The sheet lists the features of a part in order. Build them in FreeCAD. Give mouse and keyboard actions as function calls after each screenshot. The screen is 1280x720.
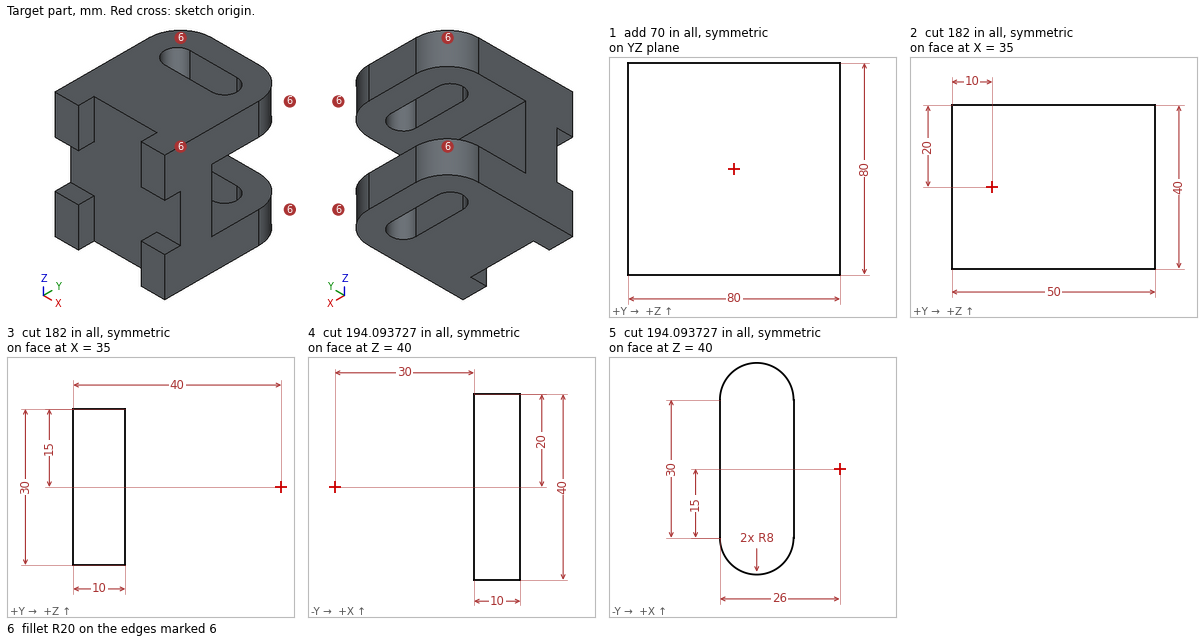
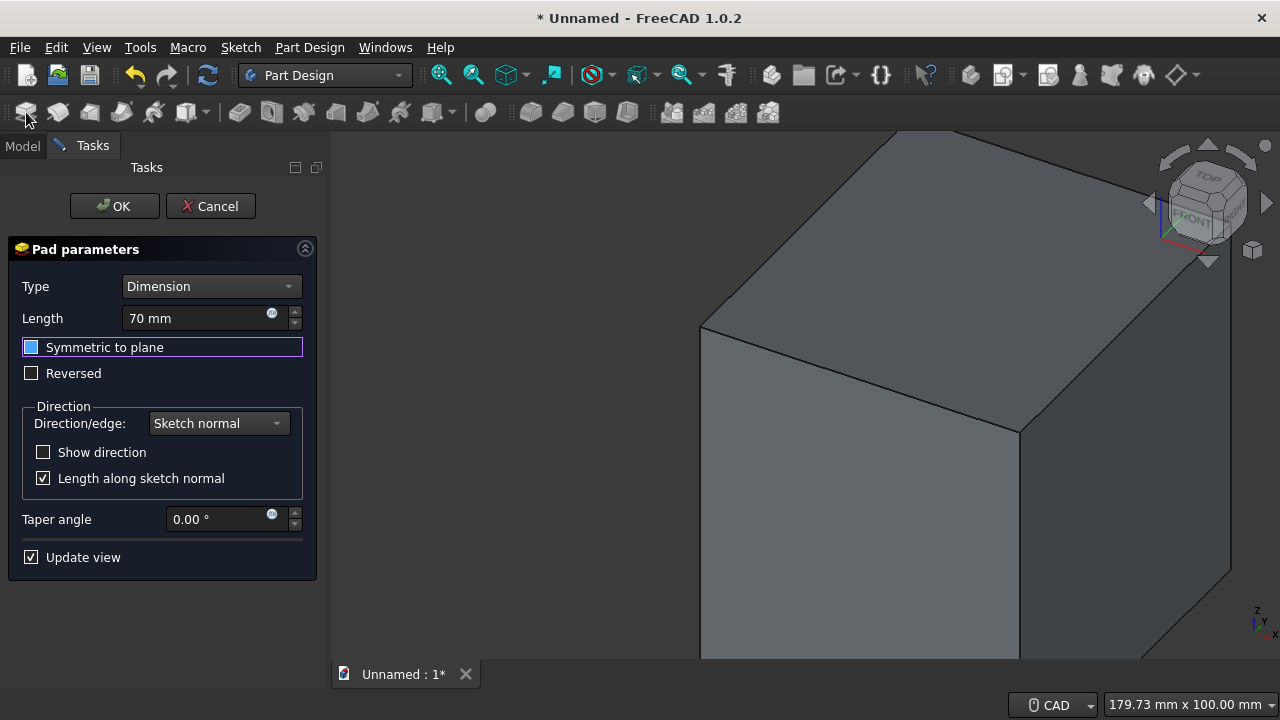
click(30, 347)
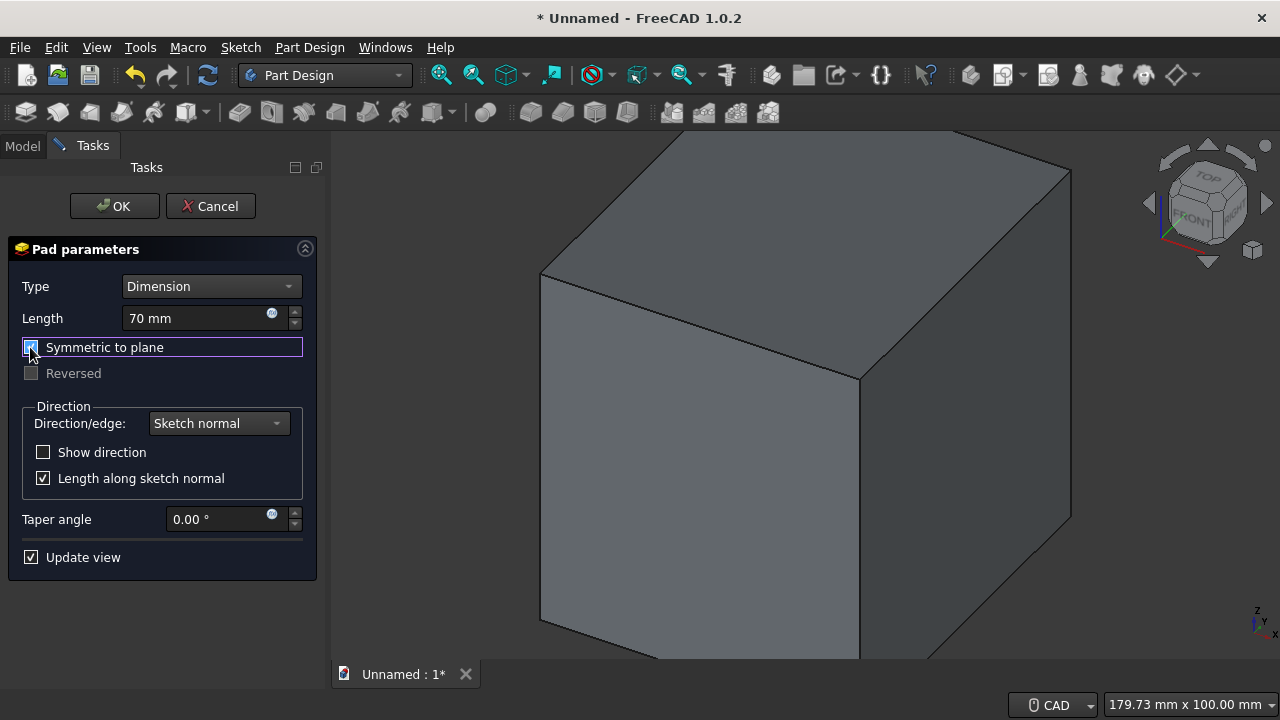
click(115, 206)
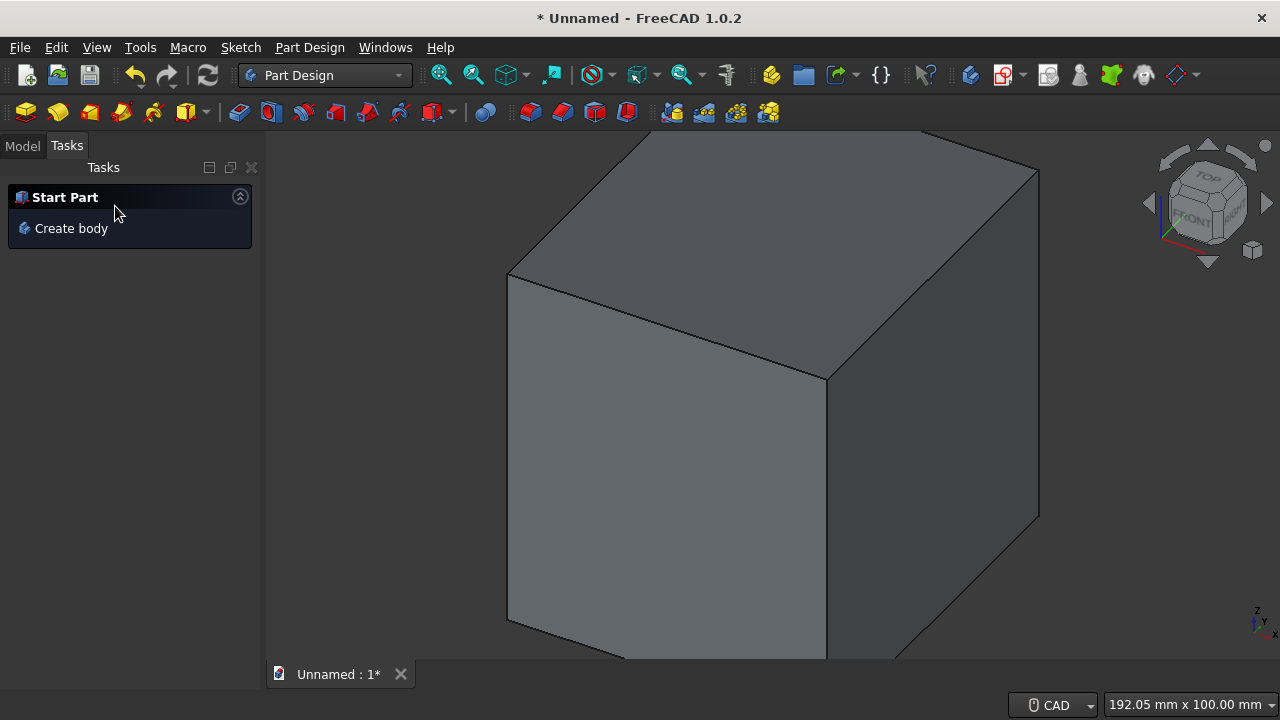
click(442, 76)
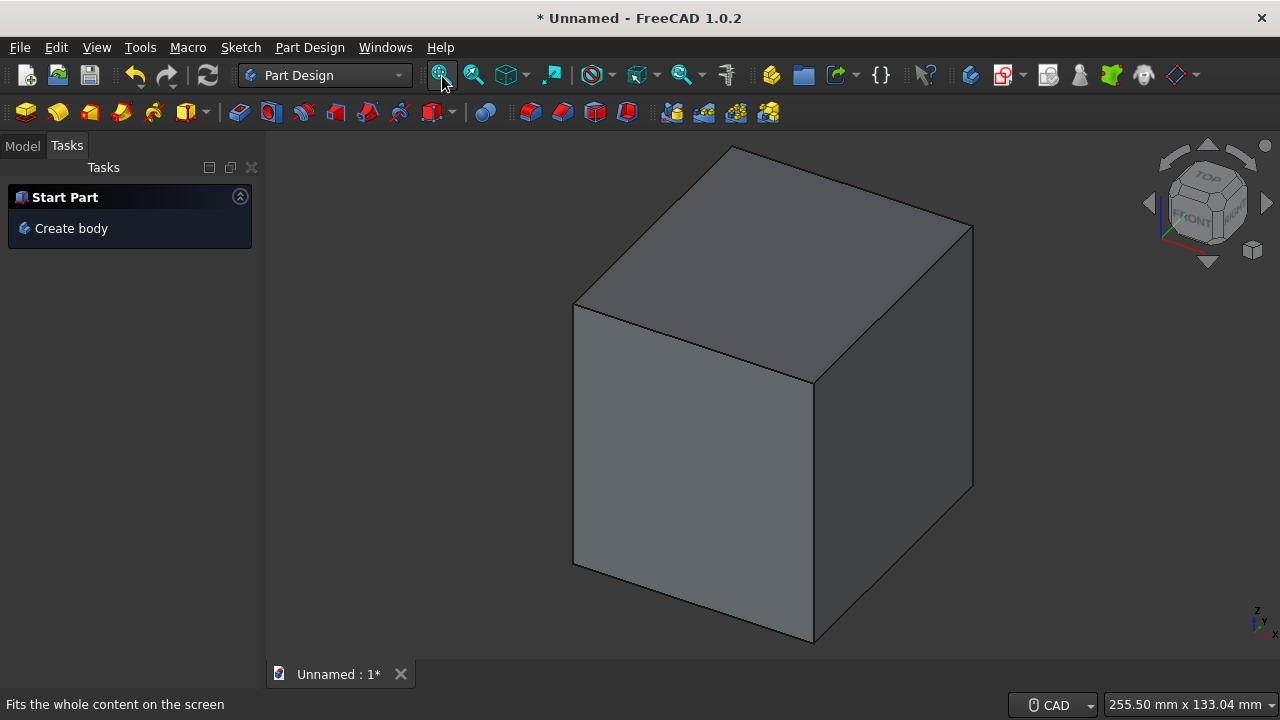
click(893, 434)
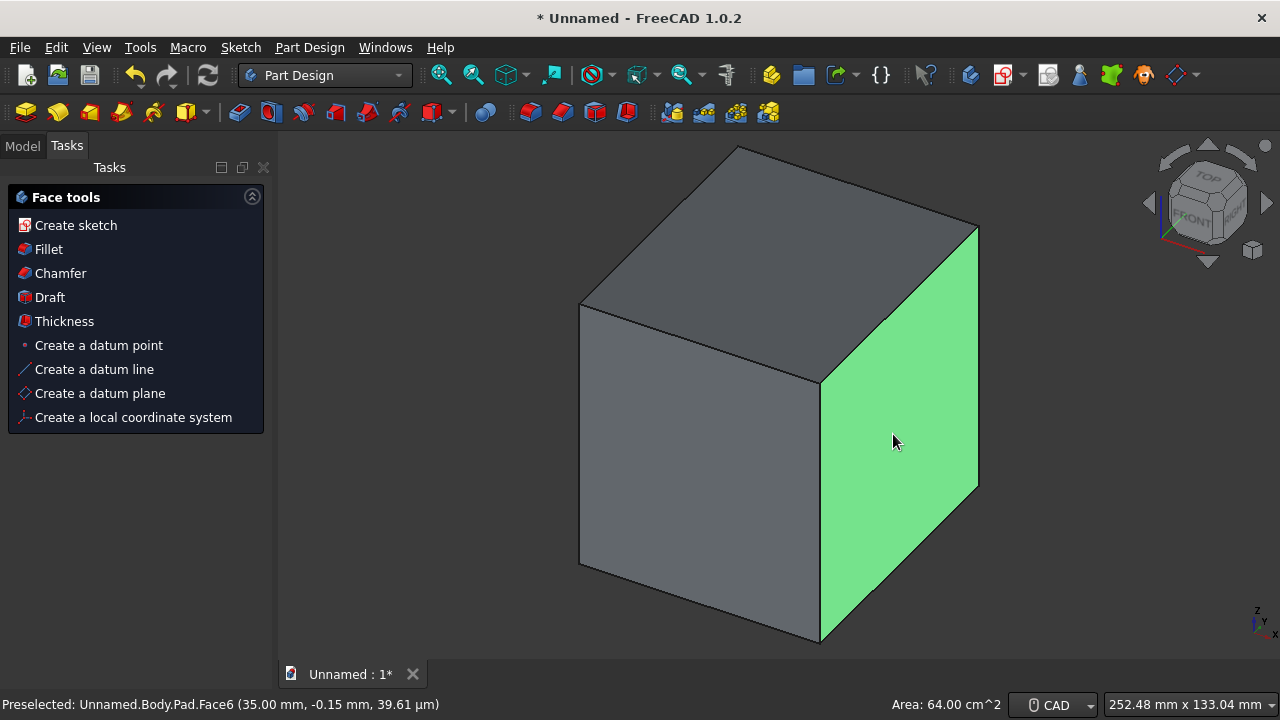
click(1004, 76)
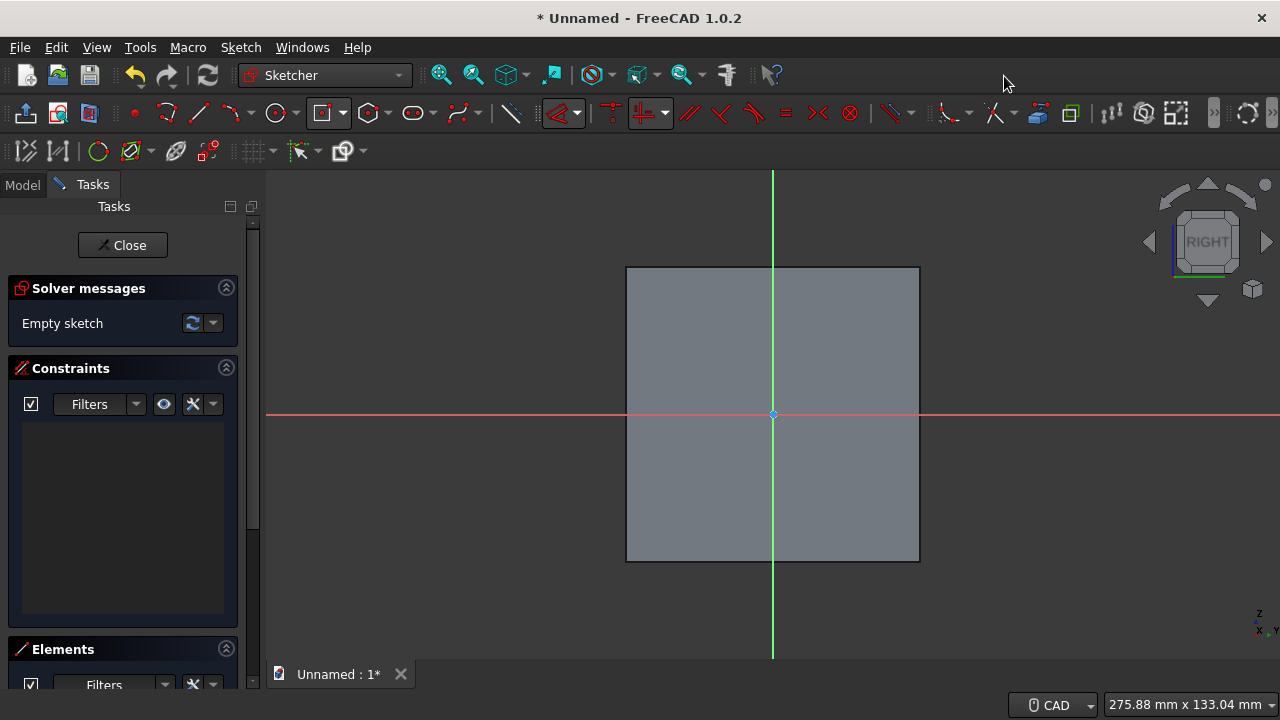
scroll(929, 414, up, 4)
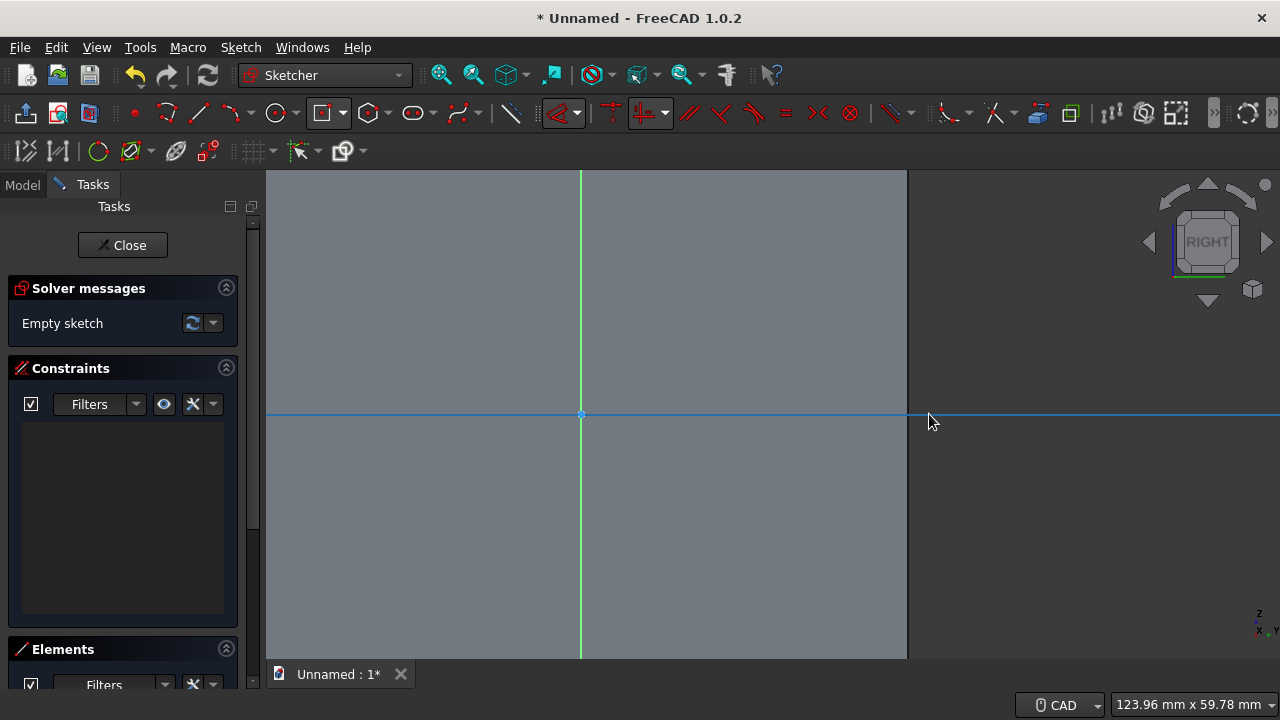
click(346, 114)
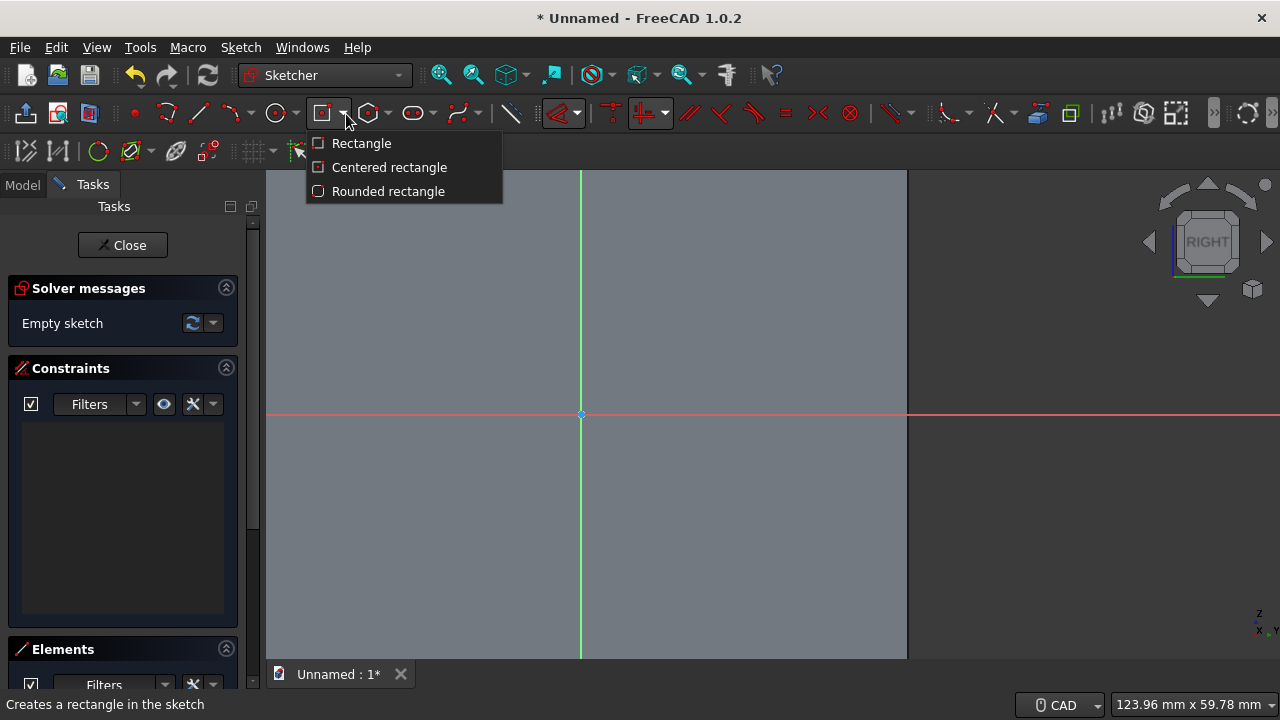
click(404, 143)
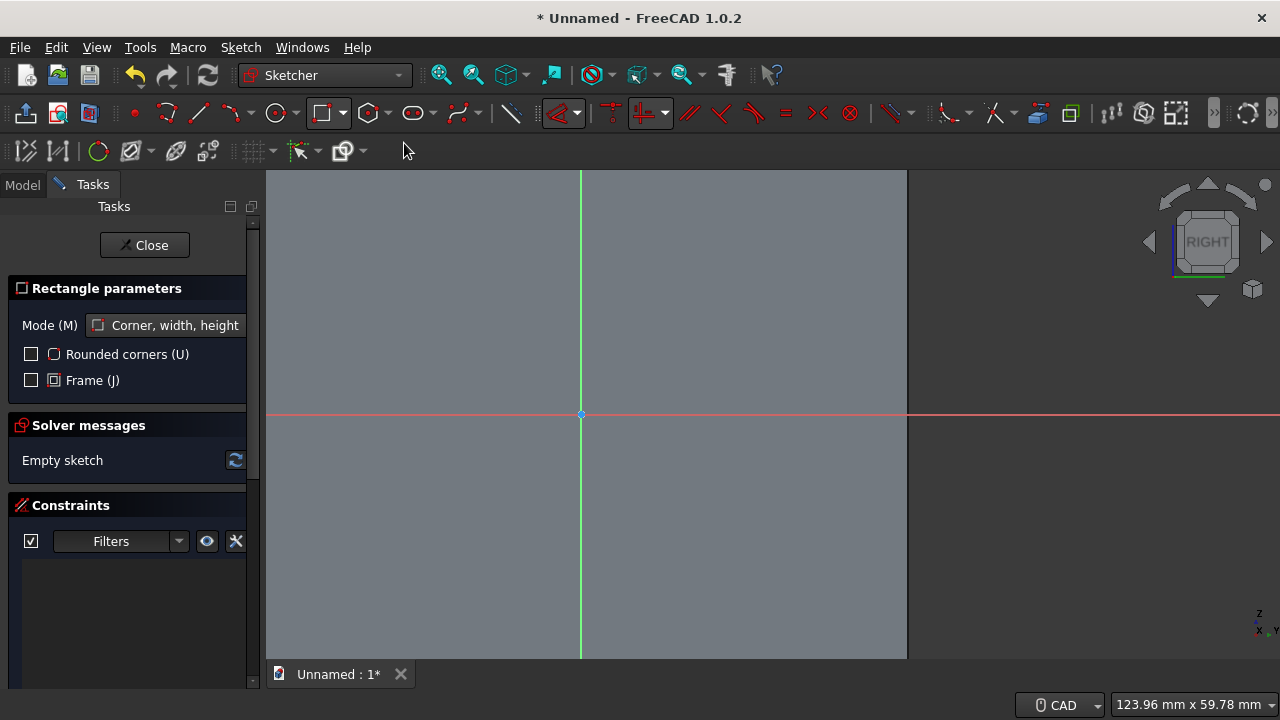
click(499, 251)
move(908, 578)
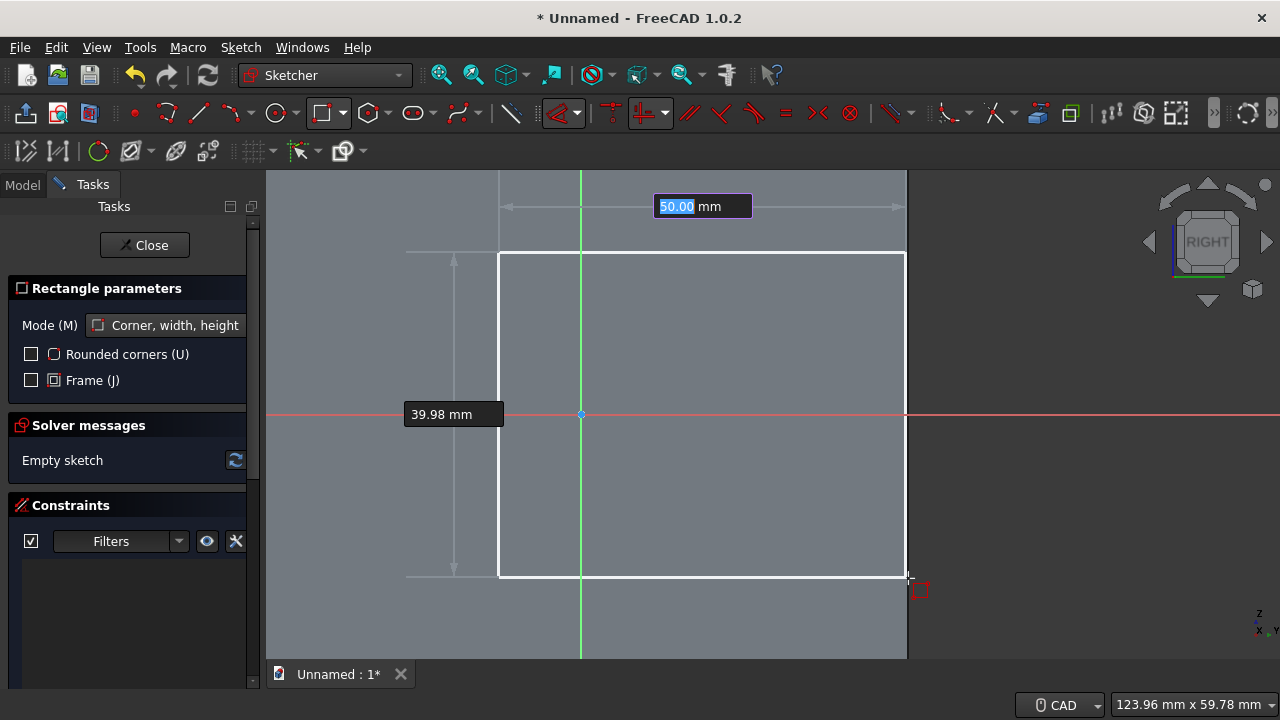
text(50)
key(Tab)
text(40)
key(Return)
key(Escape)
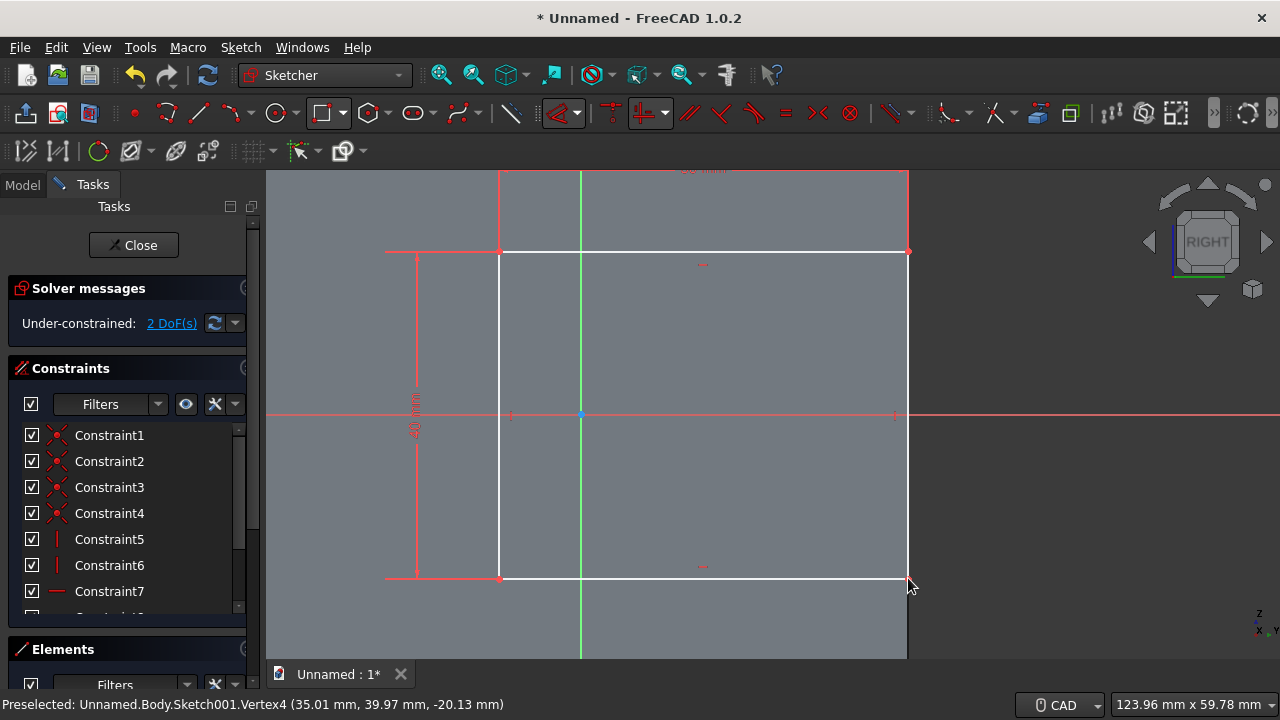
key(d)